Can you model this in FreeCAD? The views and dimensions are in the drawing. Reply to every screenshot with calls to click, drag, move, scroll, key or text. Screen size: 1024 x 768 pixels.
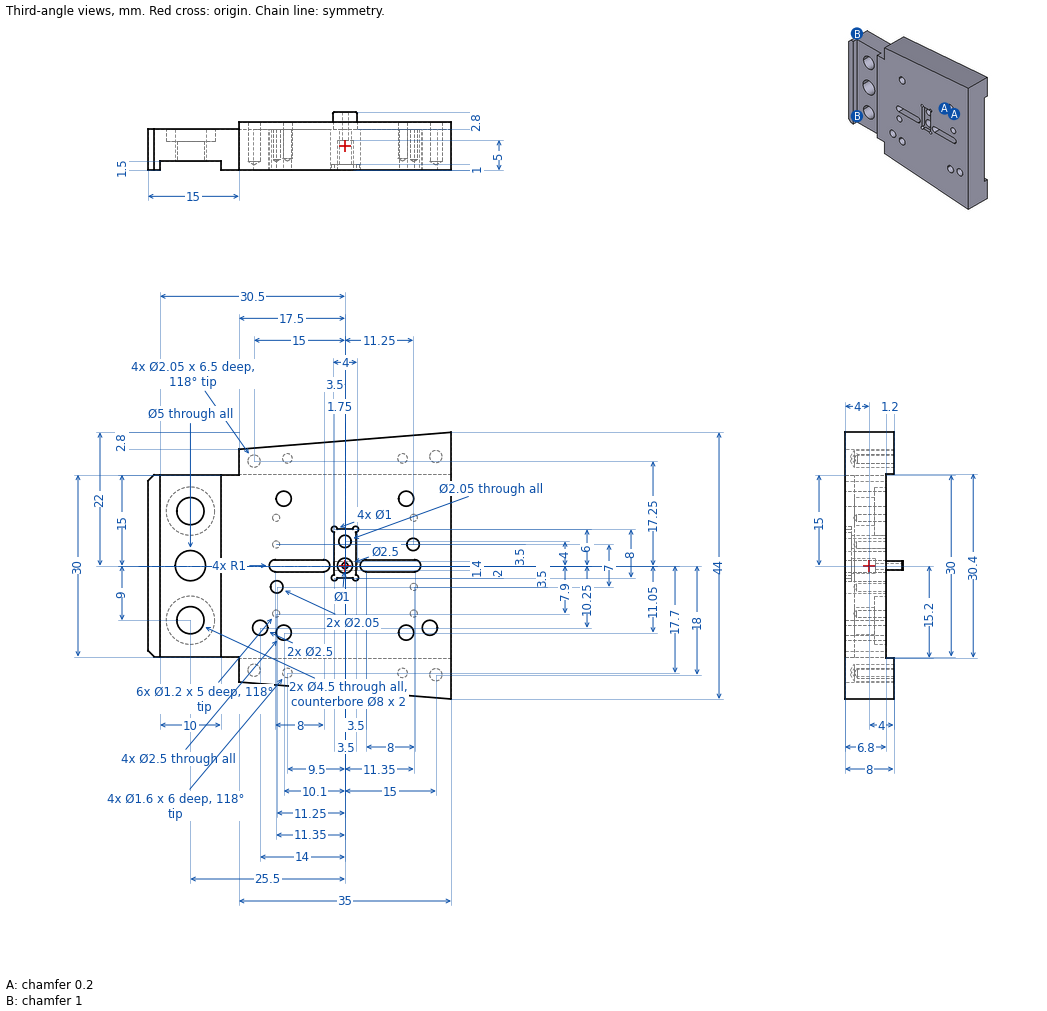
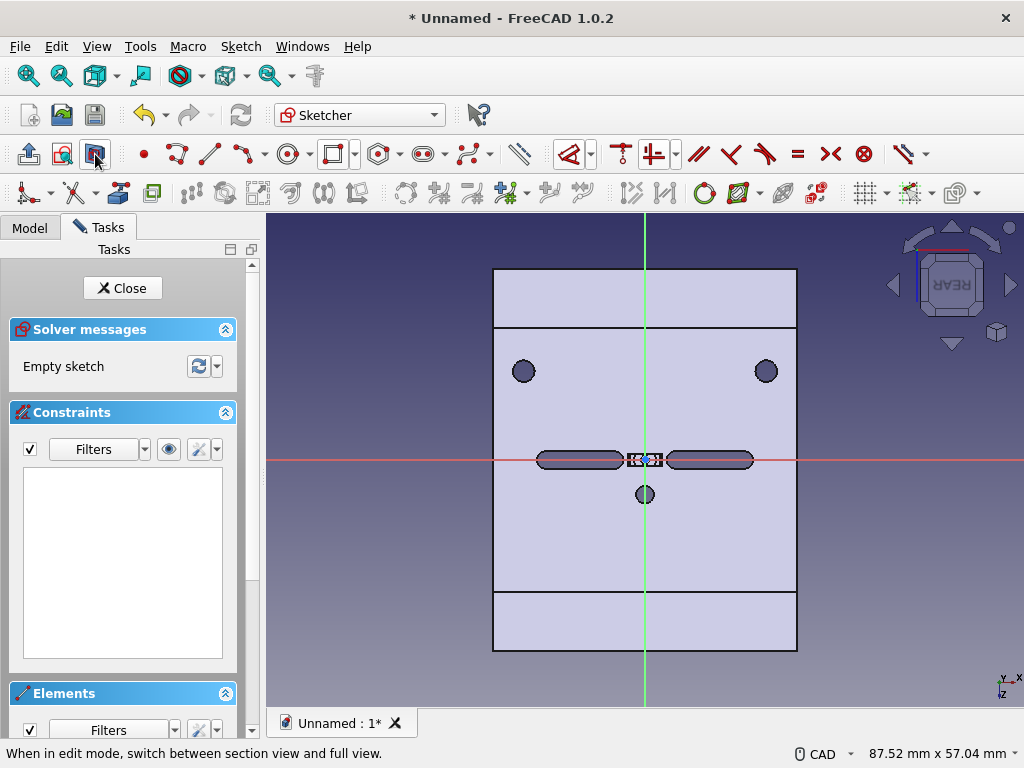
scroll(728, 460, up, 3)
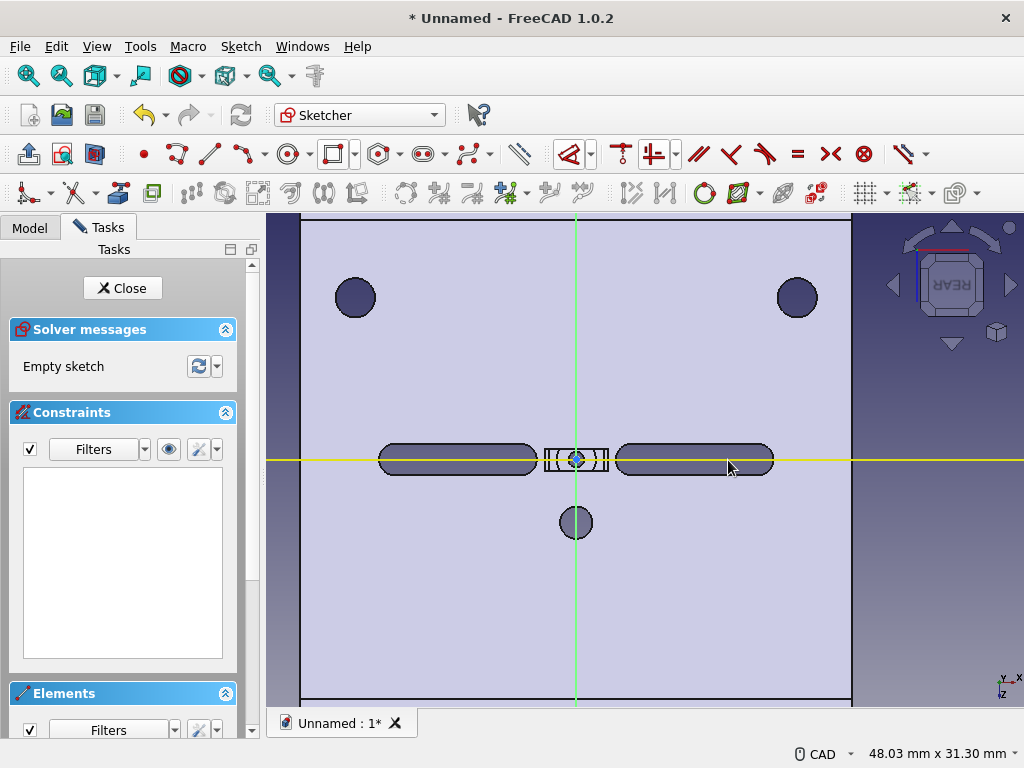
click(288, 154)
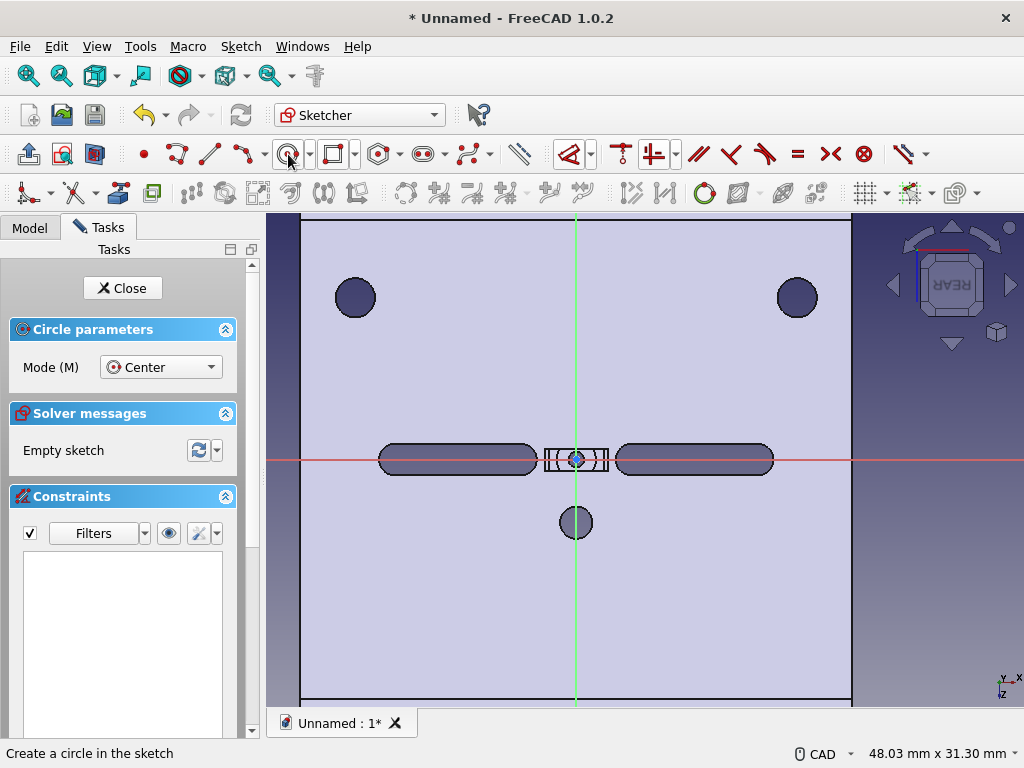
scroll(397, 335, up, 5)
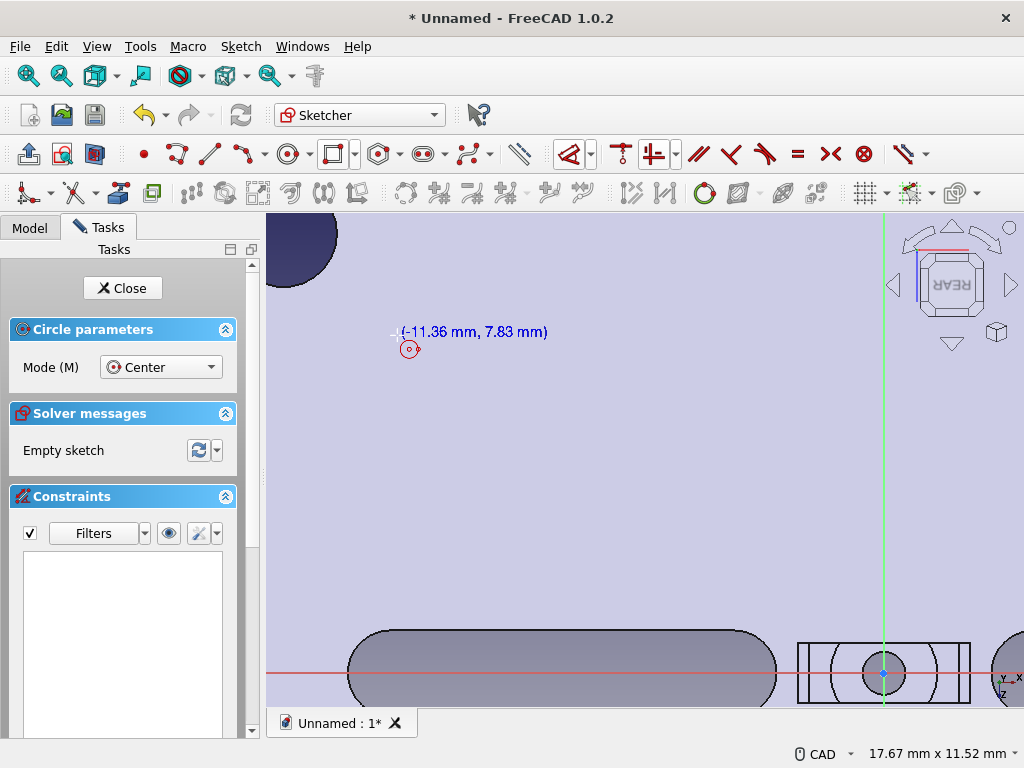
click(397, 334)
move(415, 316)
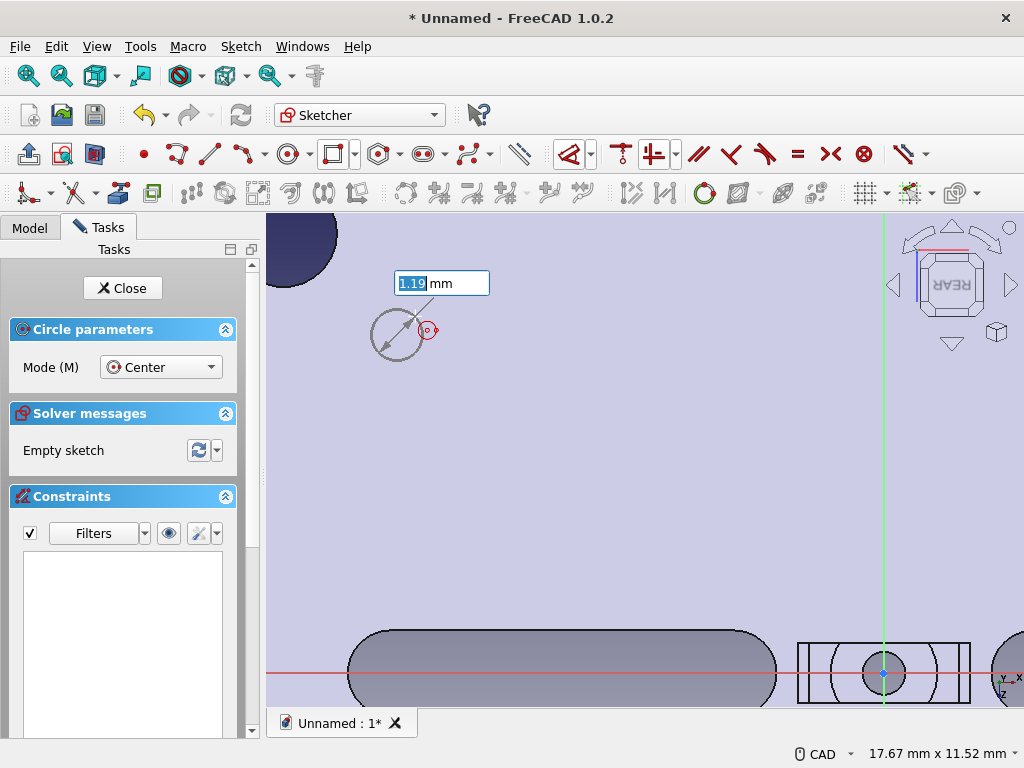
text(1.2)
key(Return)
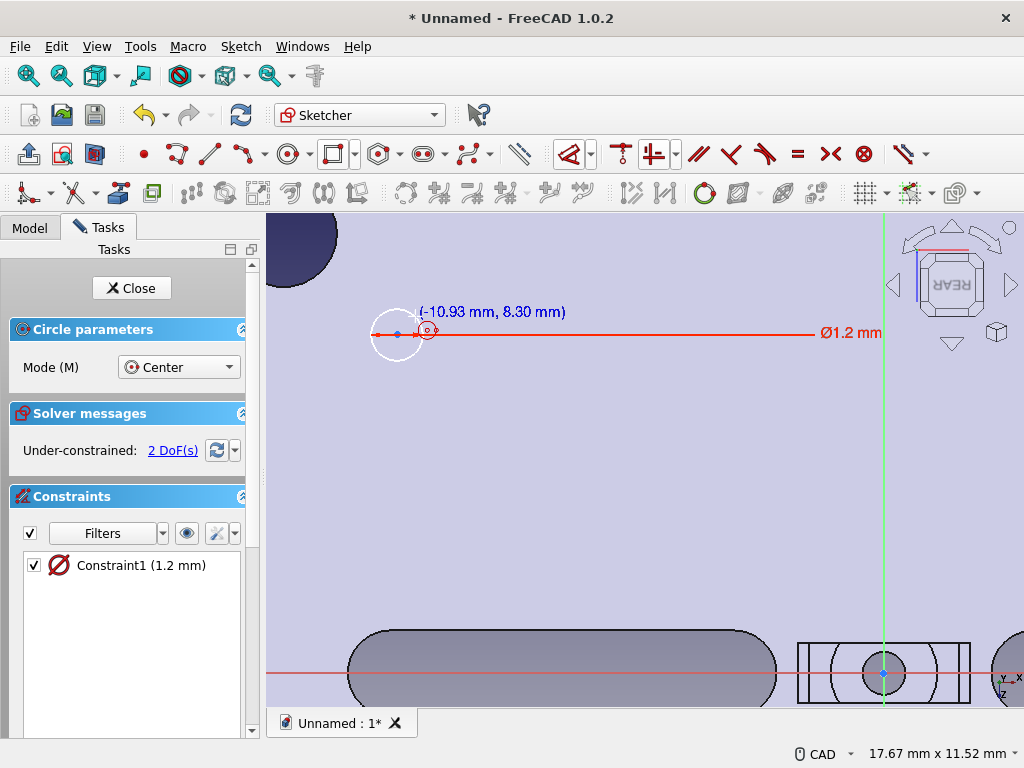
scroll(398, 336, down, 5)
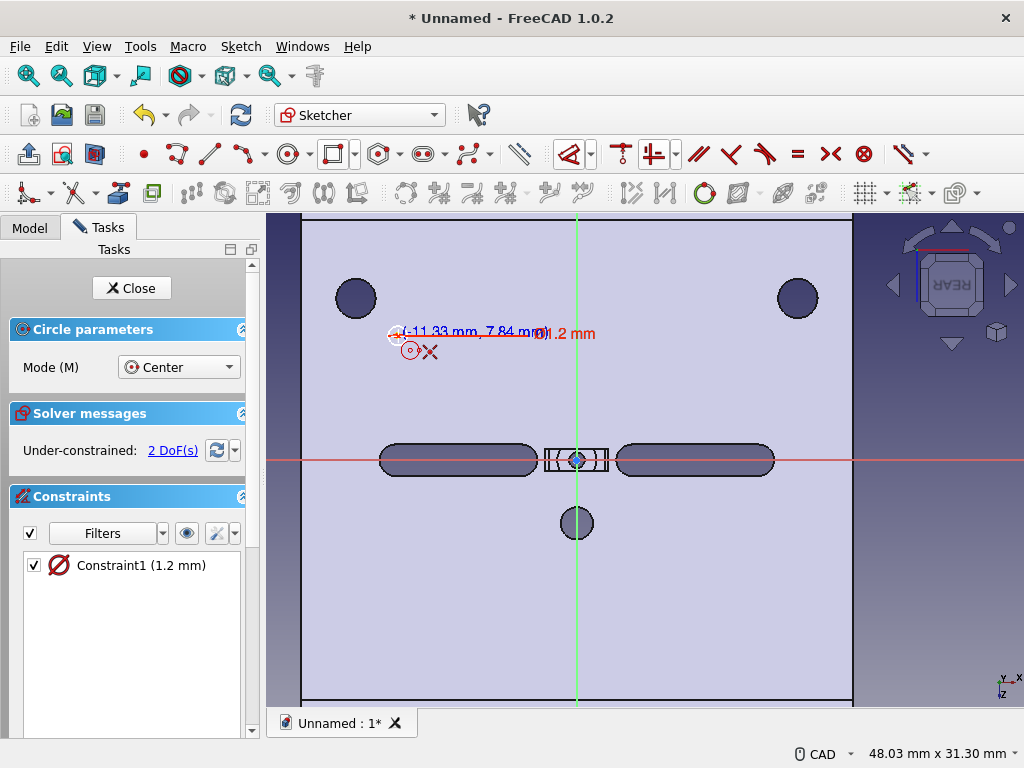
scroll(756, 336, up, 5)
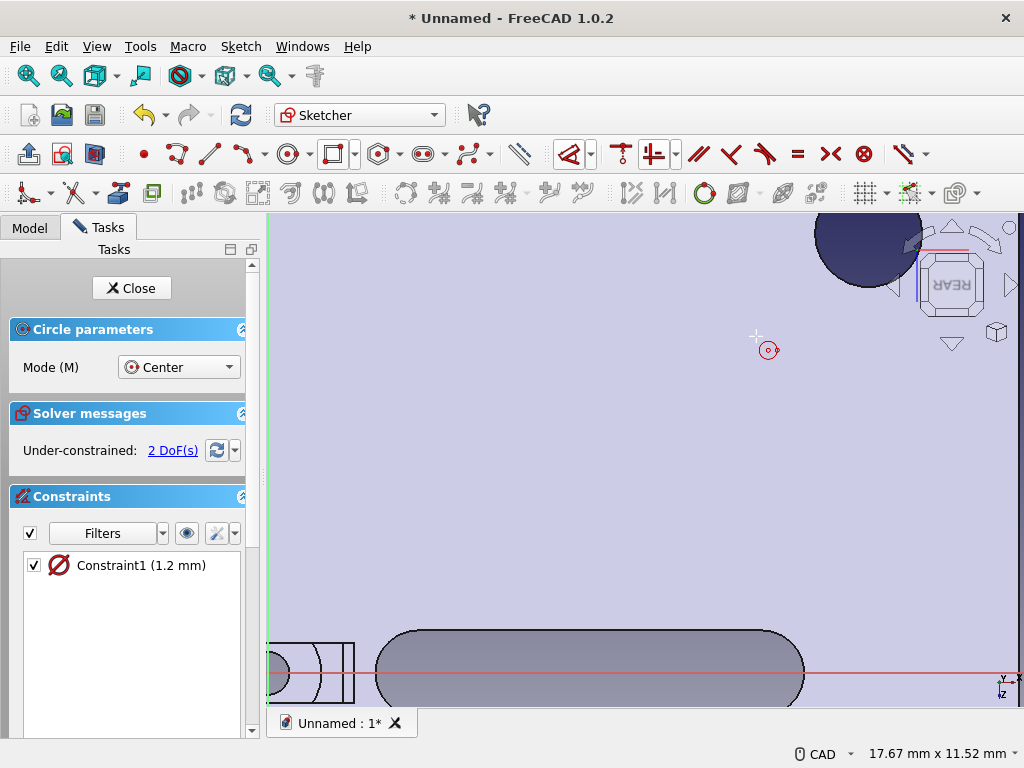
click(755, 334)
move(773, 316)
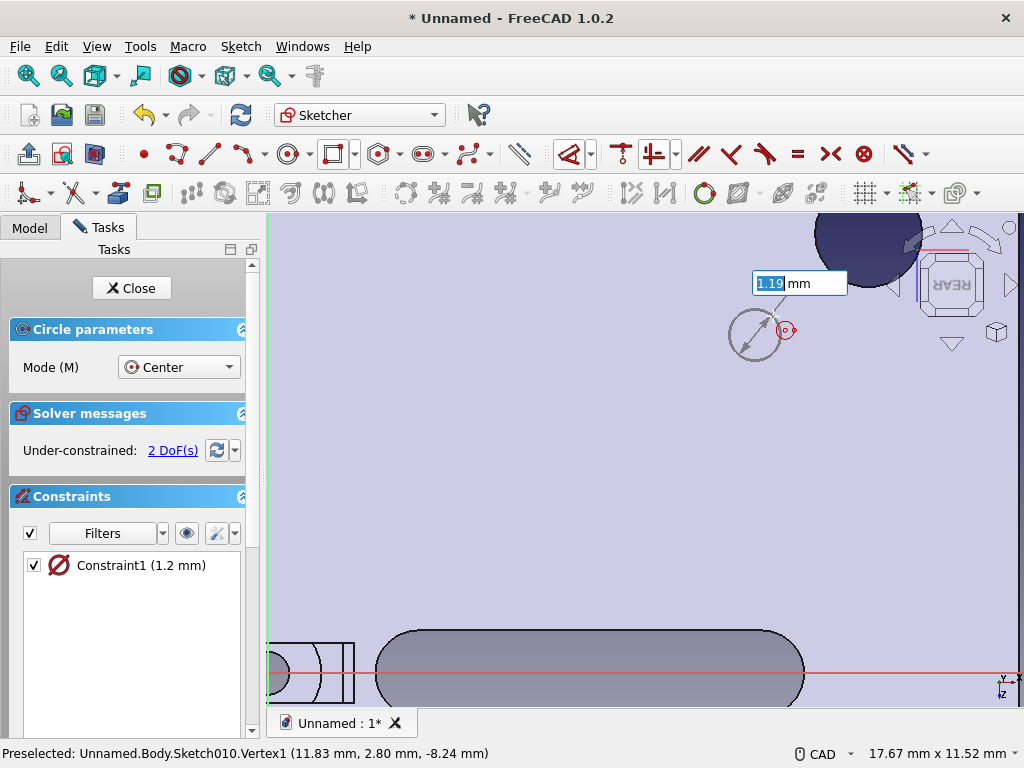
text(1.2)
key(Return)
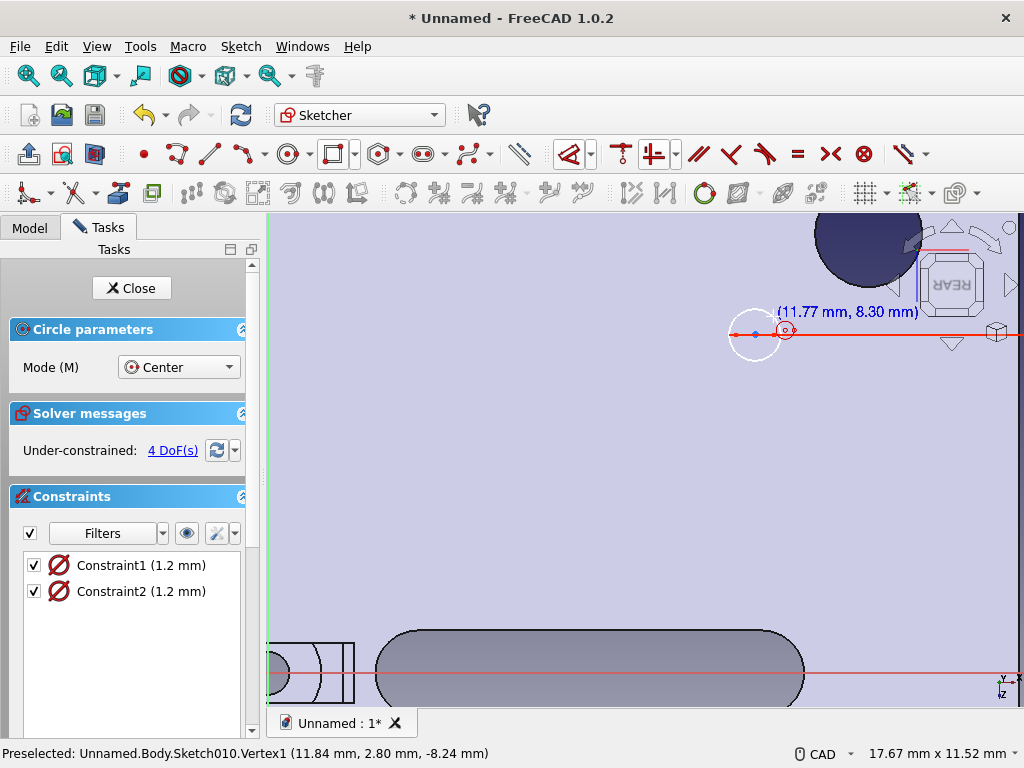
scroll(756, 336, down, 5)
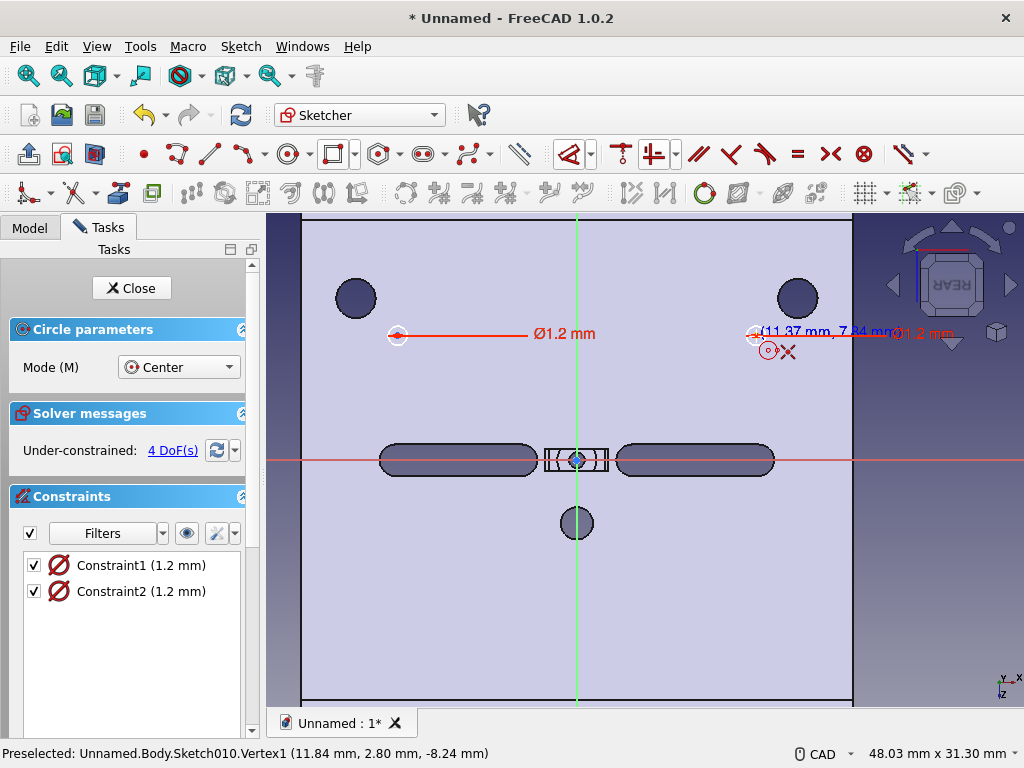
scroll(398, 515, up, 5)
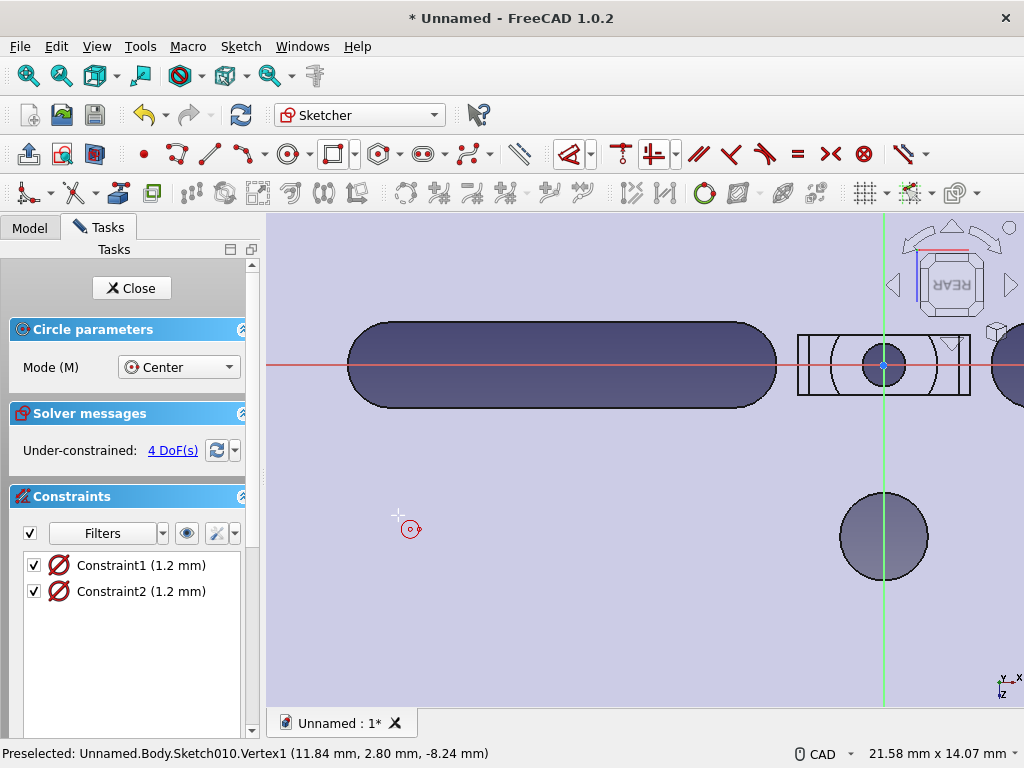
click(397, 515)
move(415, 497)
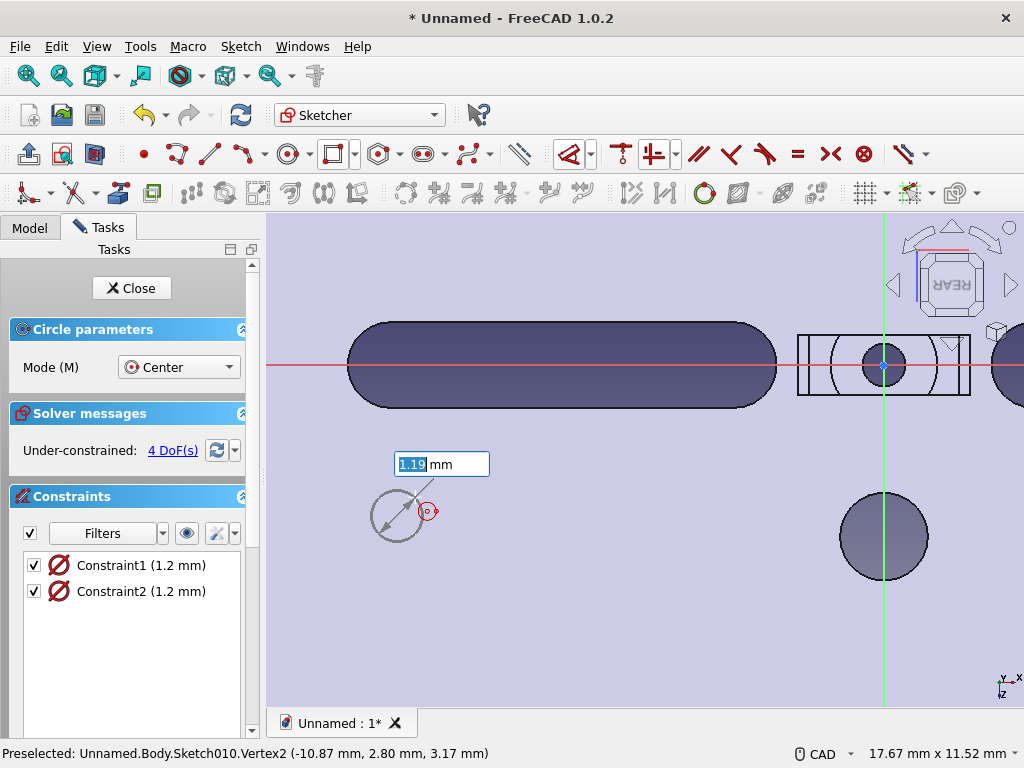
text(1.2)
key(Return)